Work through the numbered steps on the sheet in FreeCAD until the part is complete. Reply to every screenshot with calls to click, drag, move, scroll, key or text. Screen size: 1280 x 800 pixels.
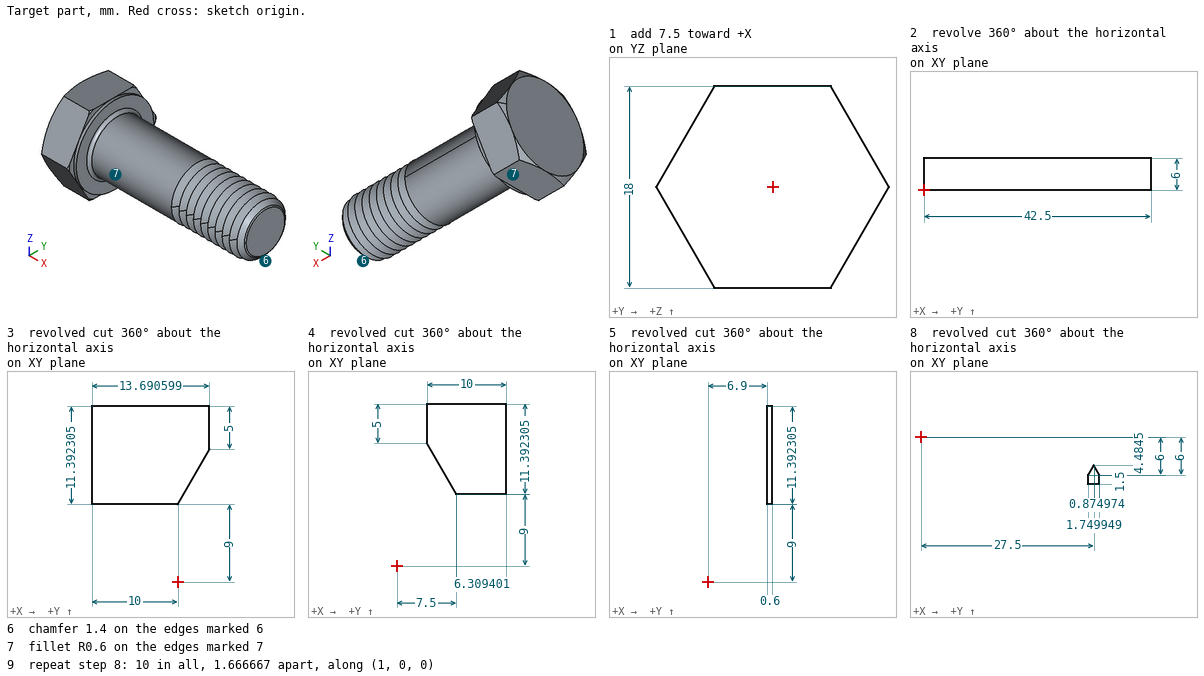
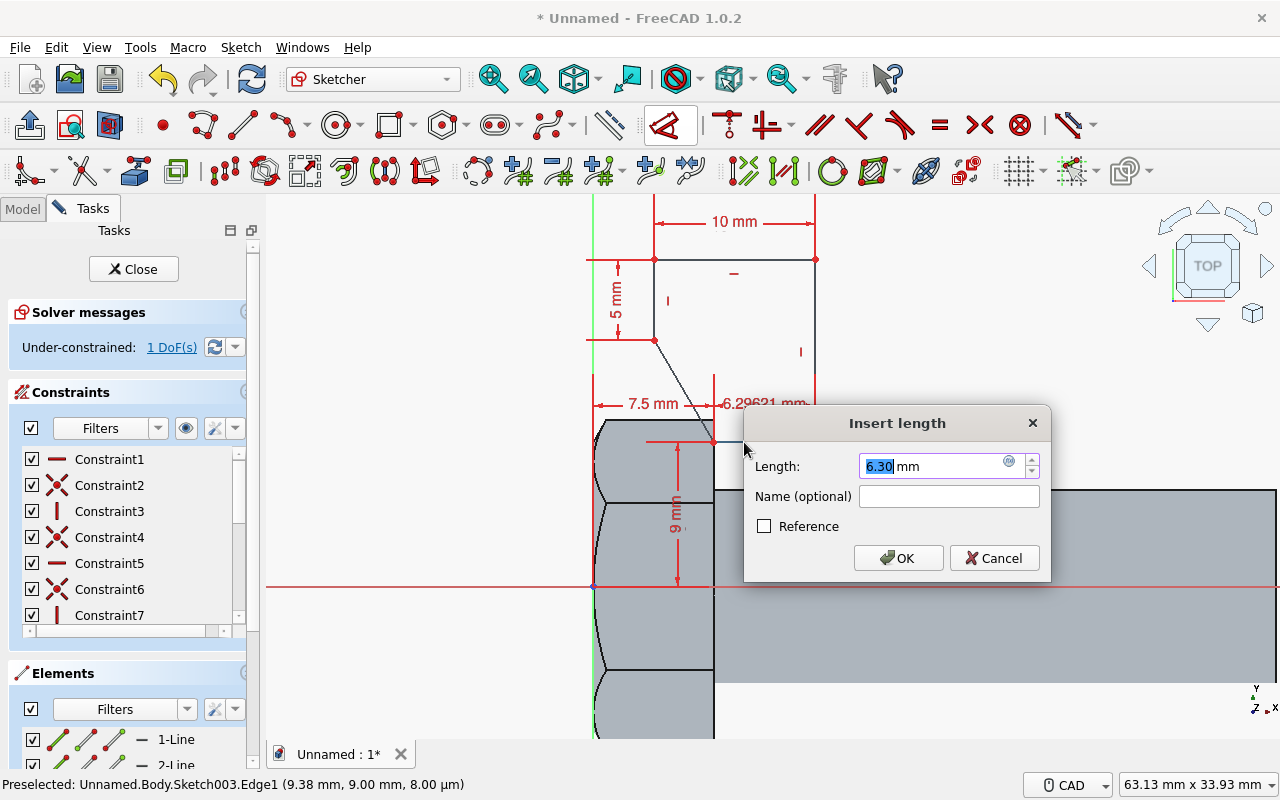
text(6.309401)
key(Return)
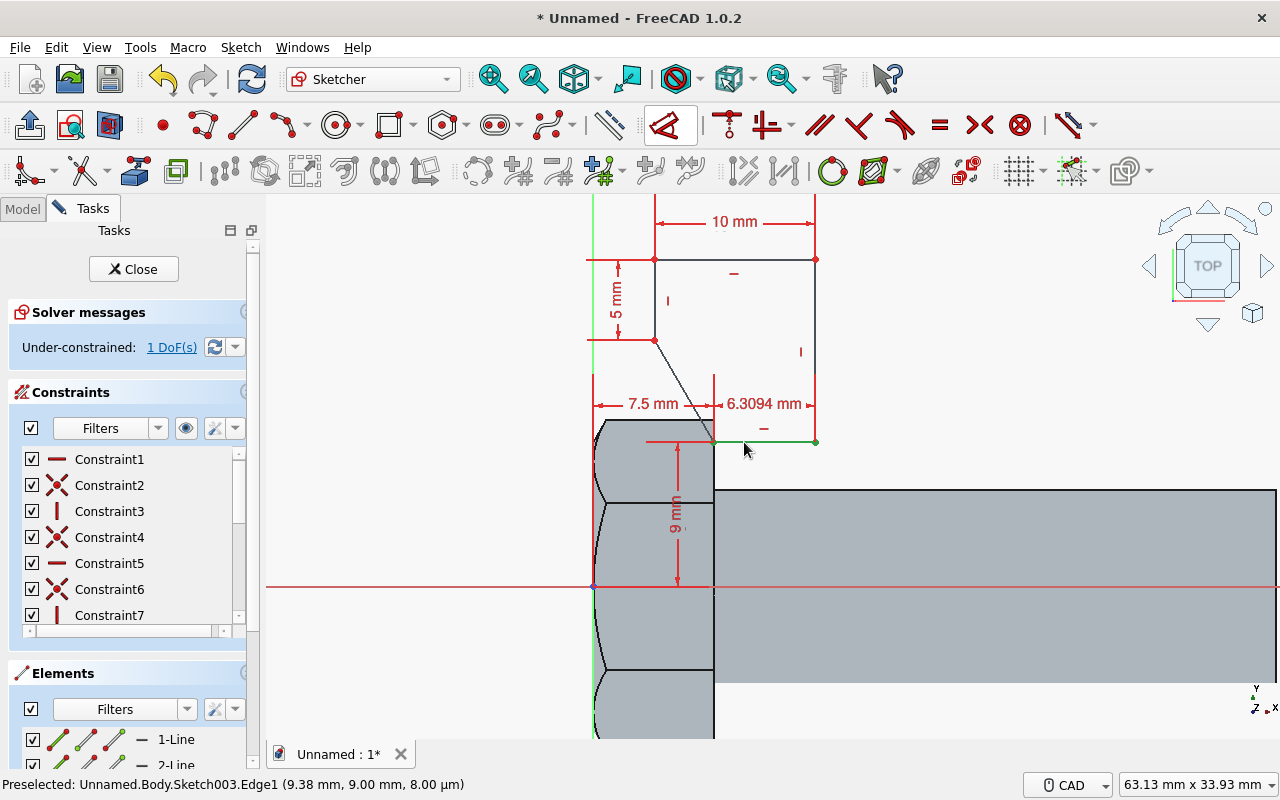
click(815, 388)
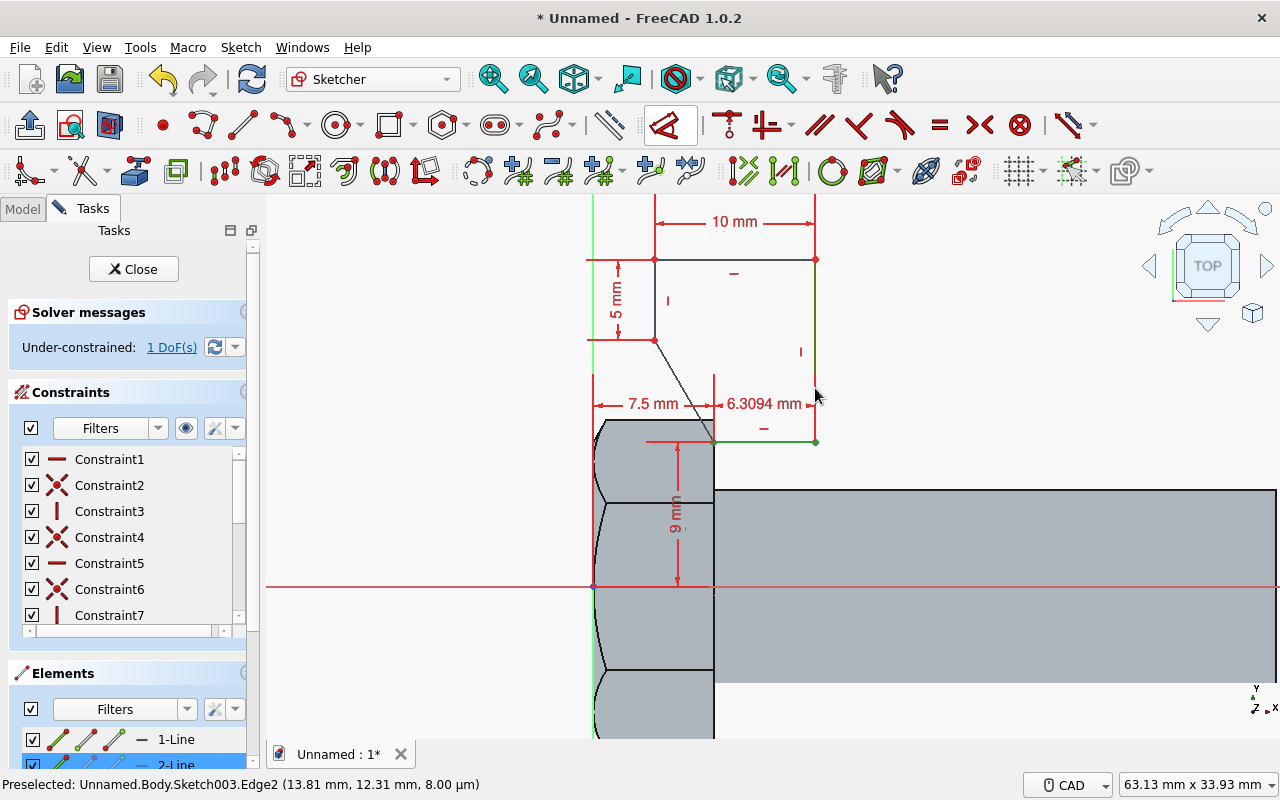
key(i)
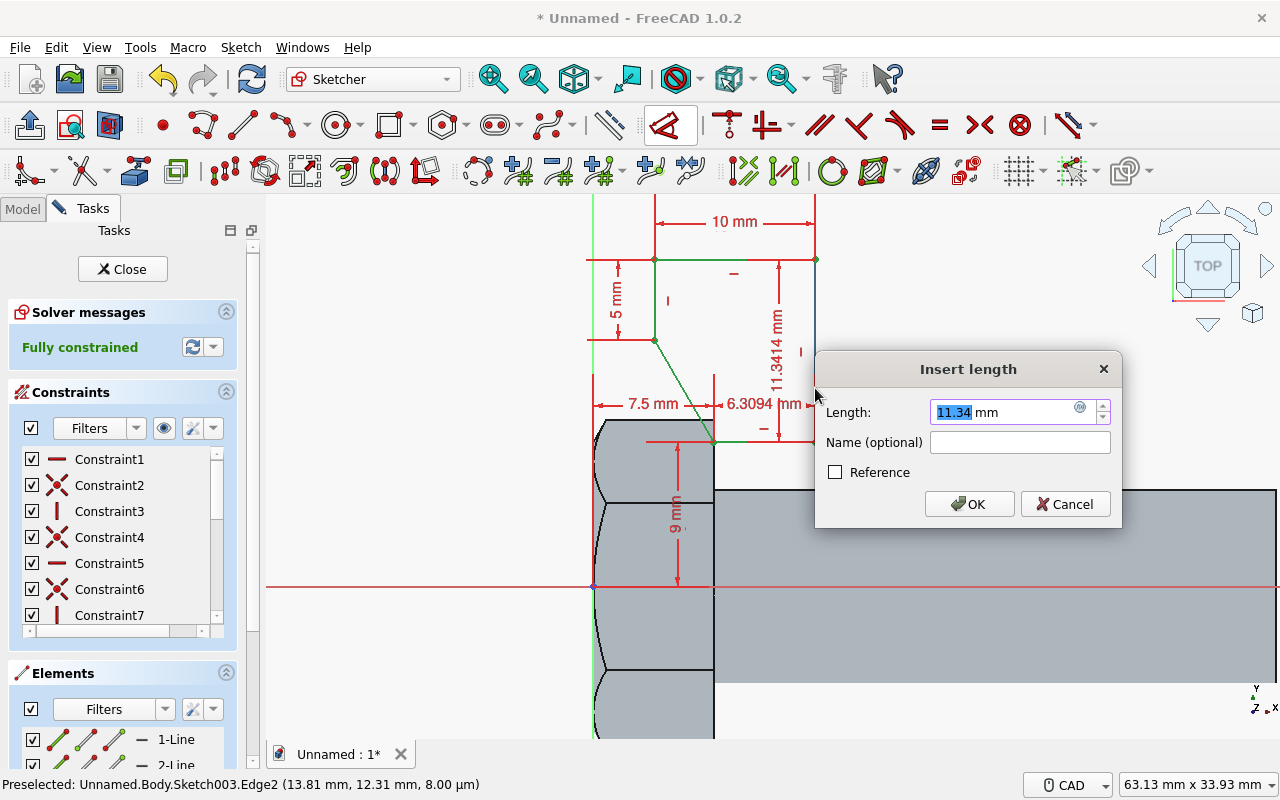
text(11.392305)
key(Return)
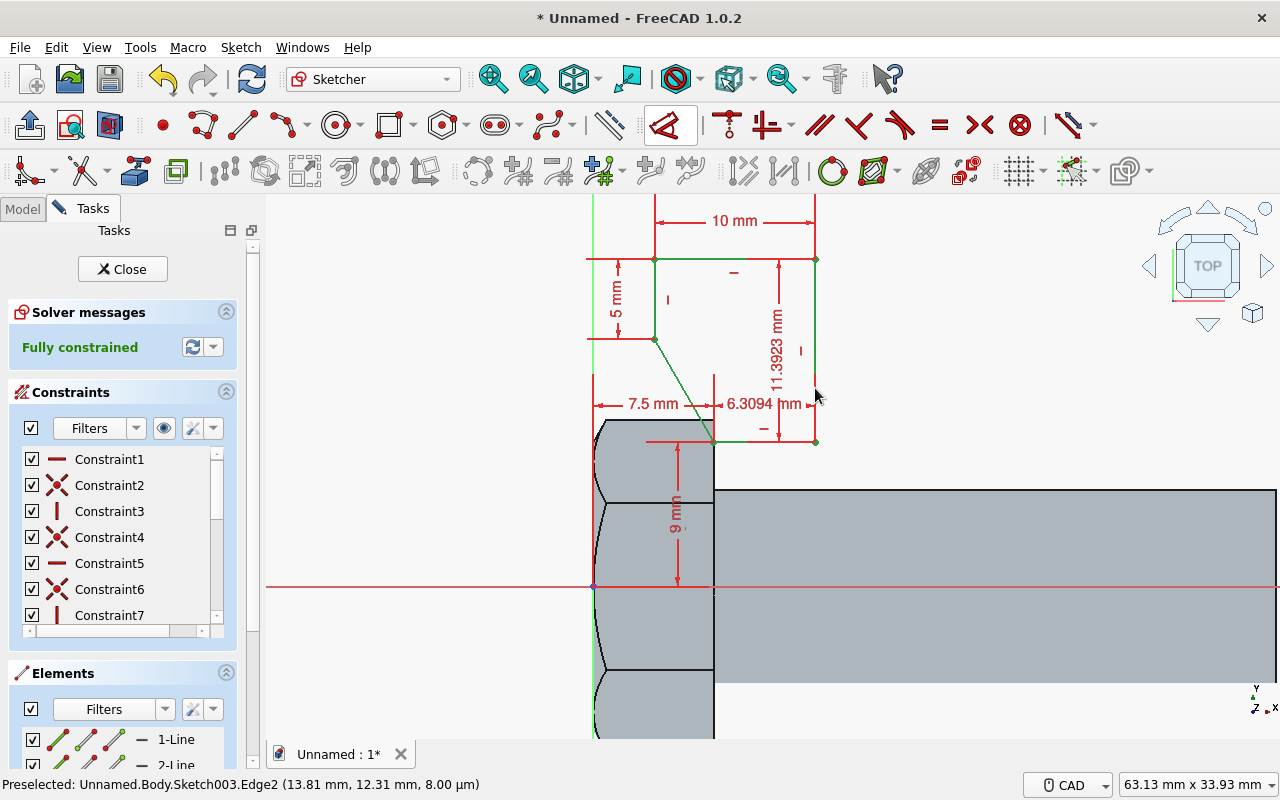
click(123, 269)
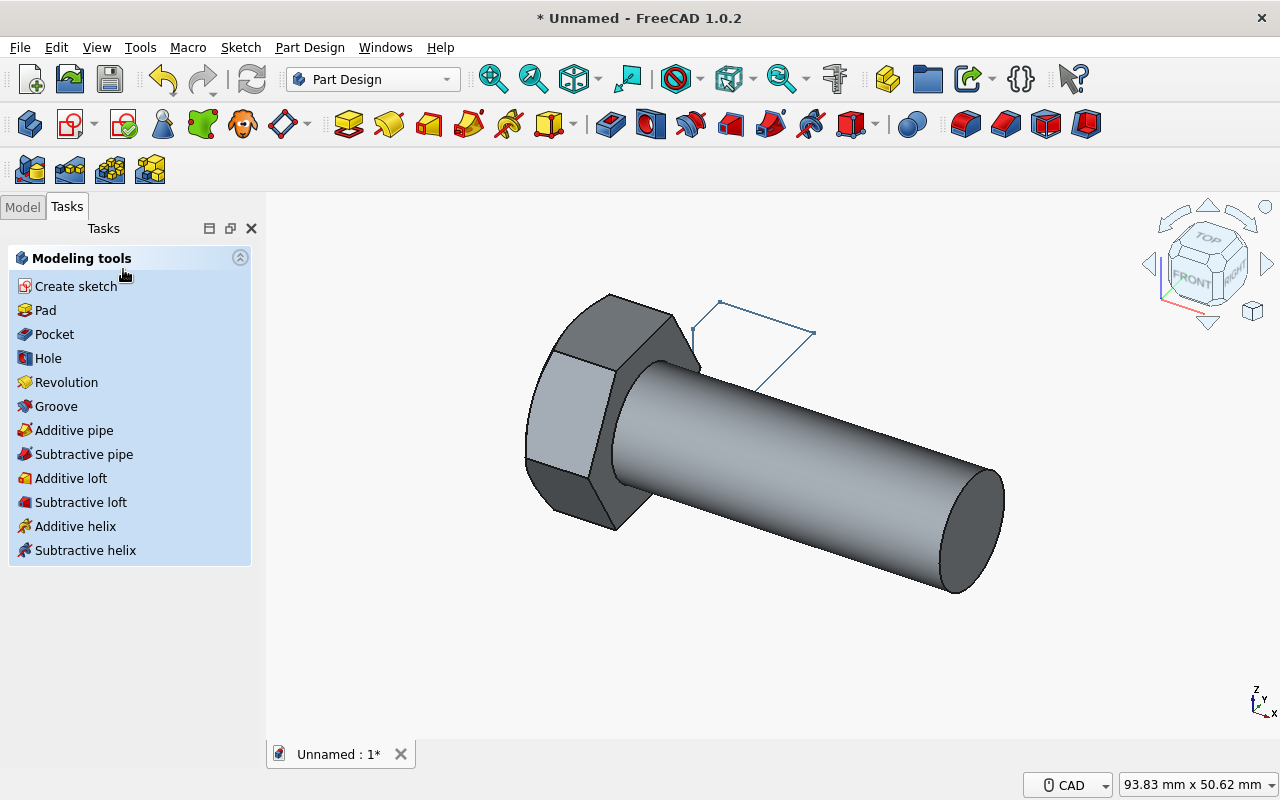
click(692, 124)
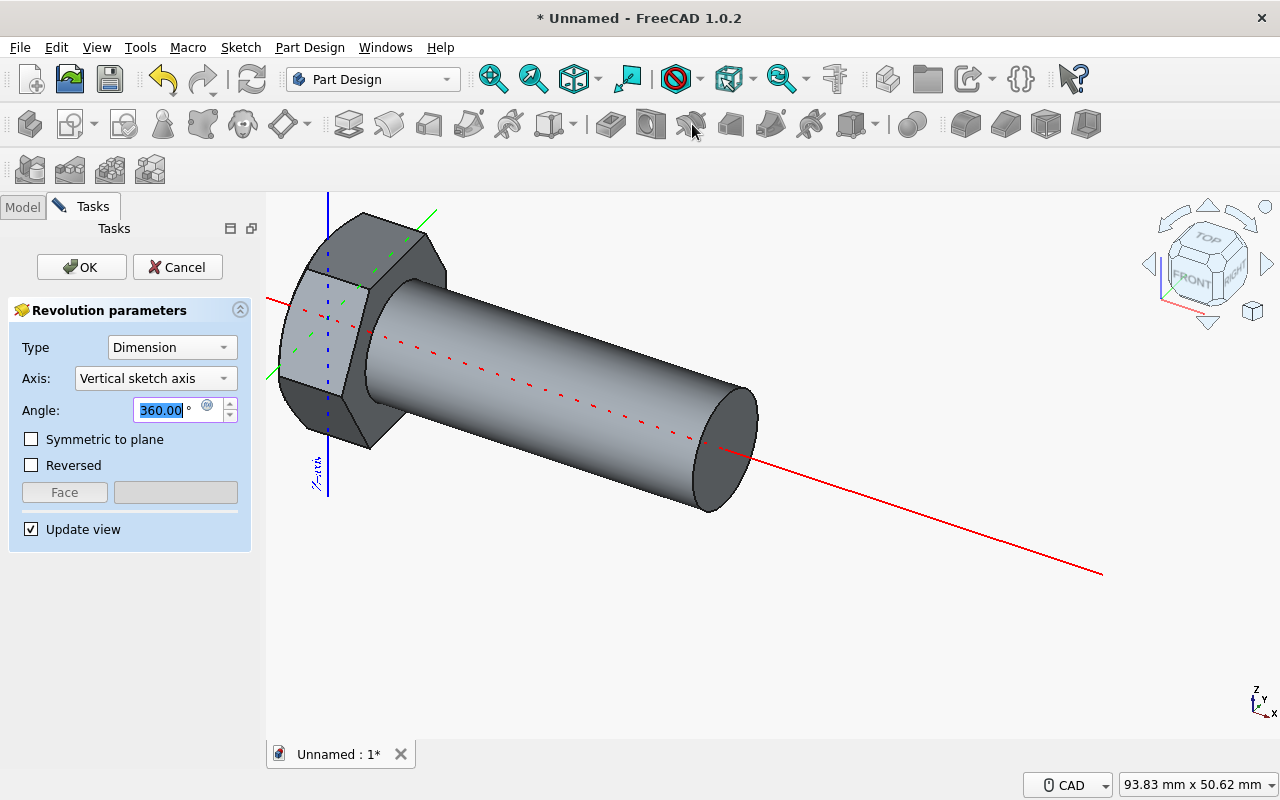
click(156, 378)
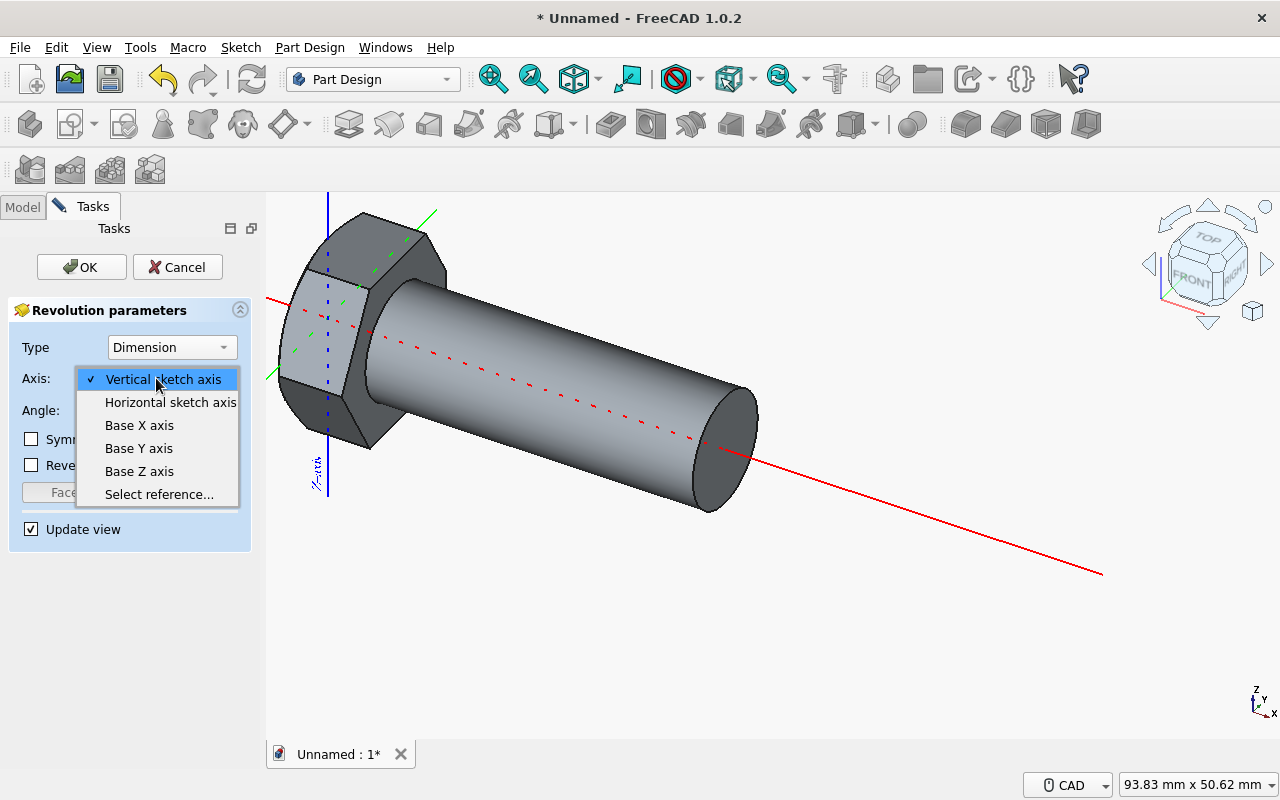
click(156, 402)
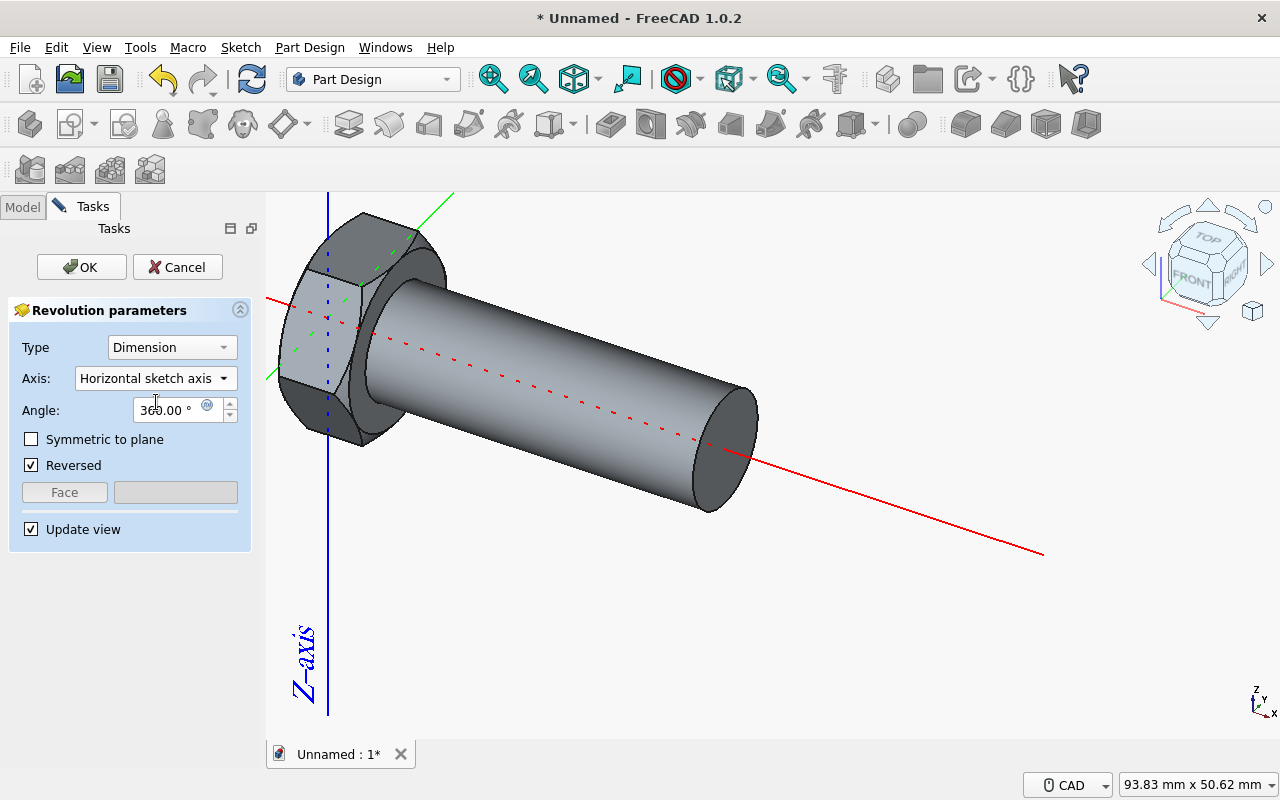
click(82, 267)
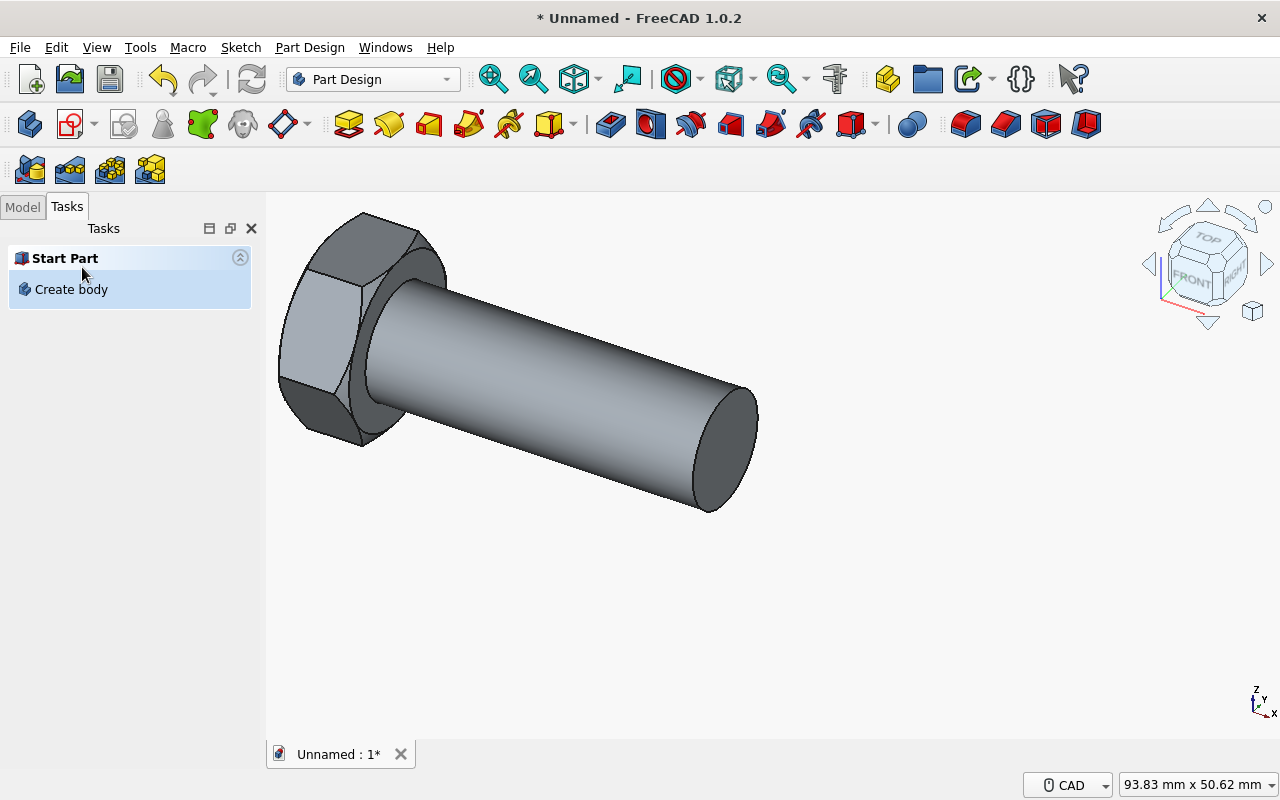
key(v)
key(f)